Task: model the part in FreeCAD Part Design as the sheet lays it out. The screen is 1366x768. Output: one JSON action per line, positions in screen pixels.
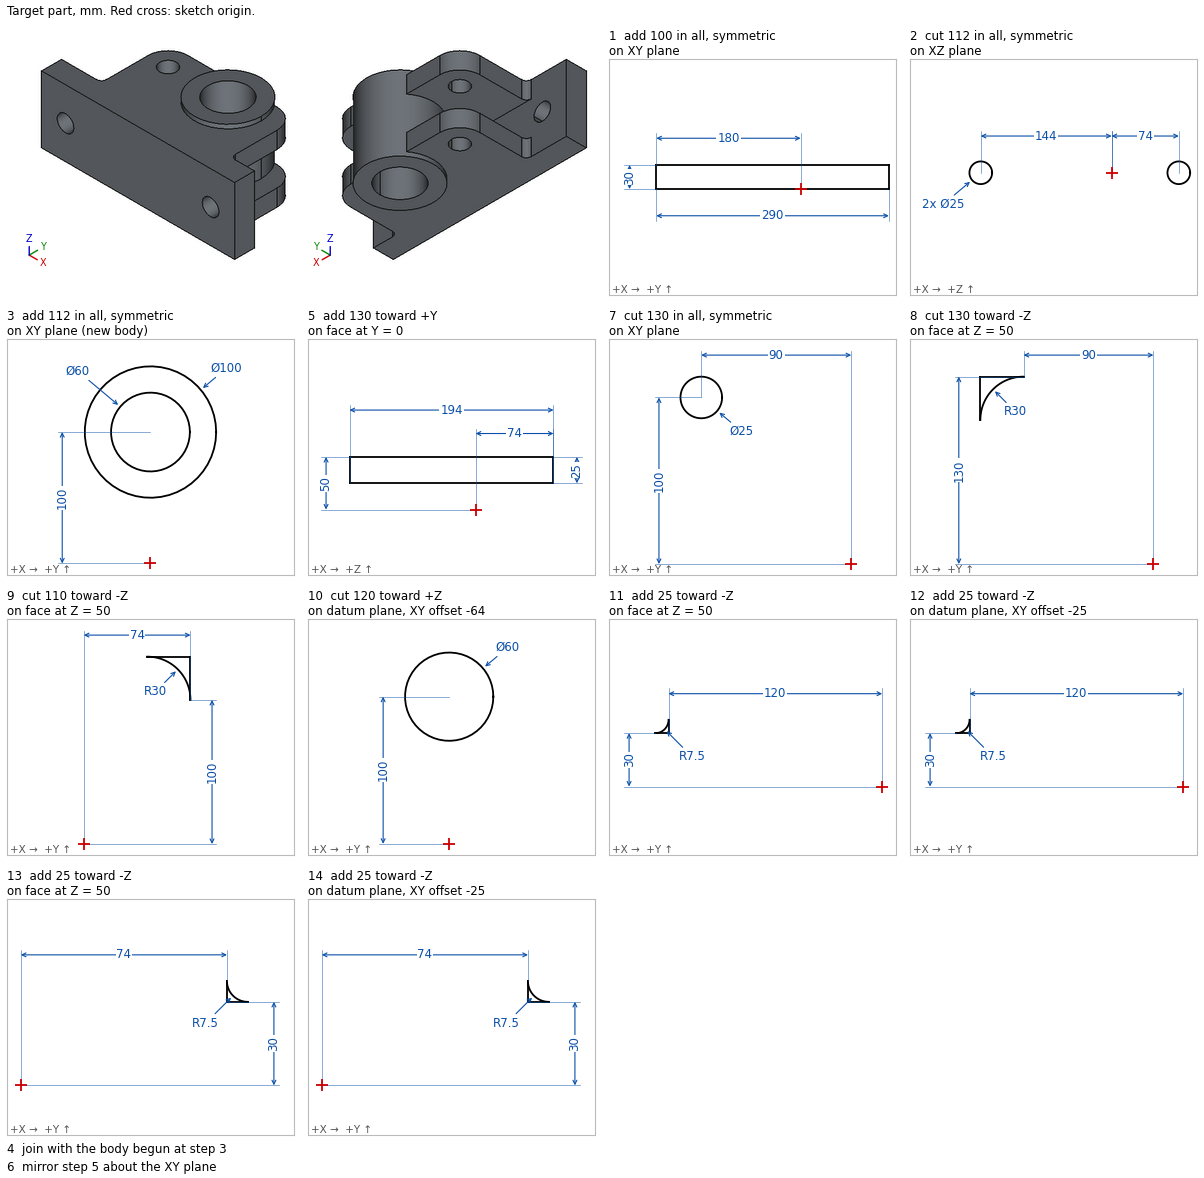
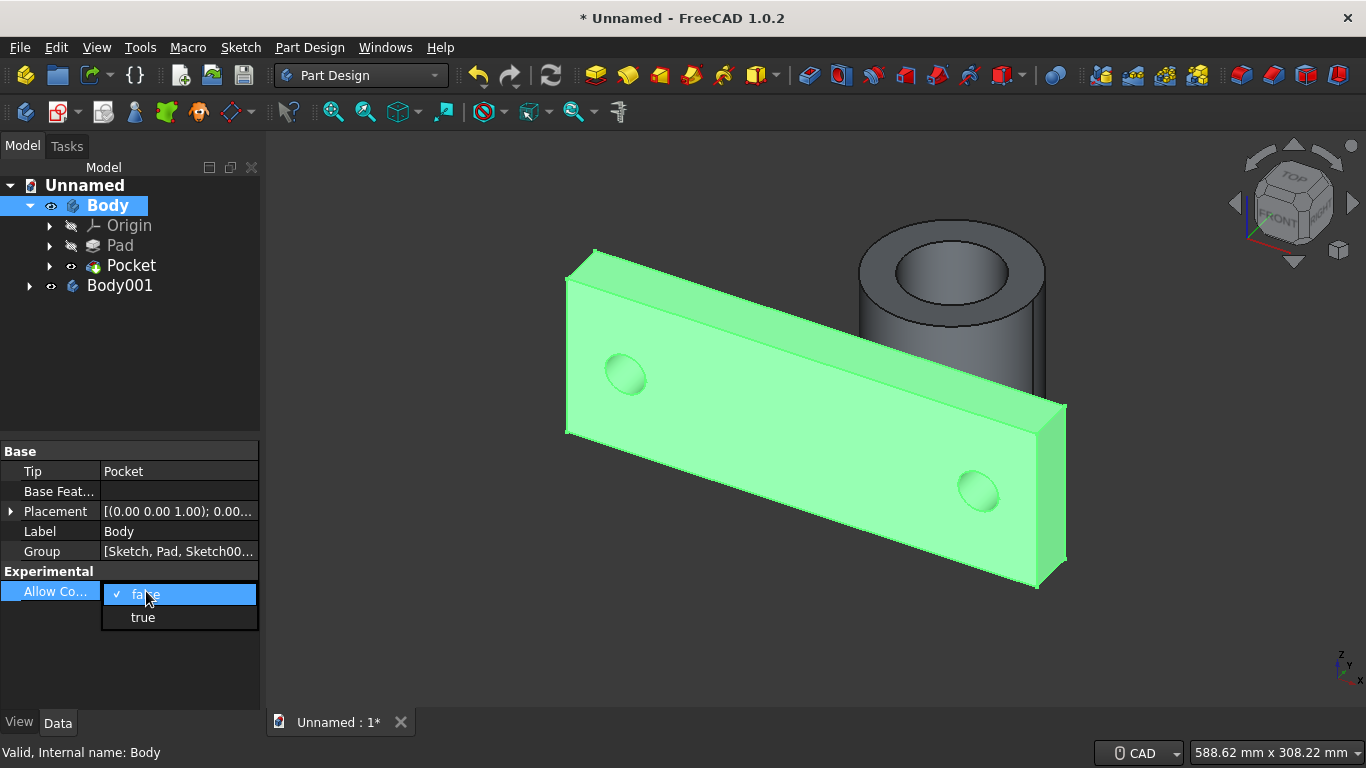
{"action": "left_click", "coordinate": [179, 618]}
{"action": "key", "text": "Return"}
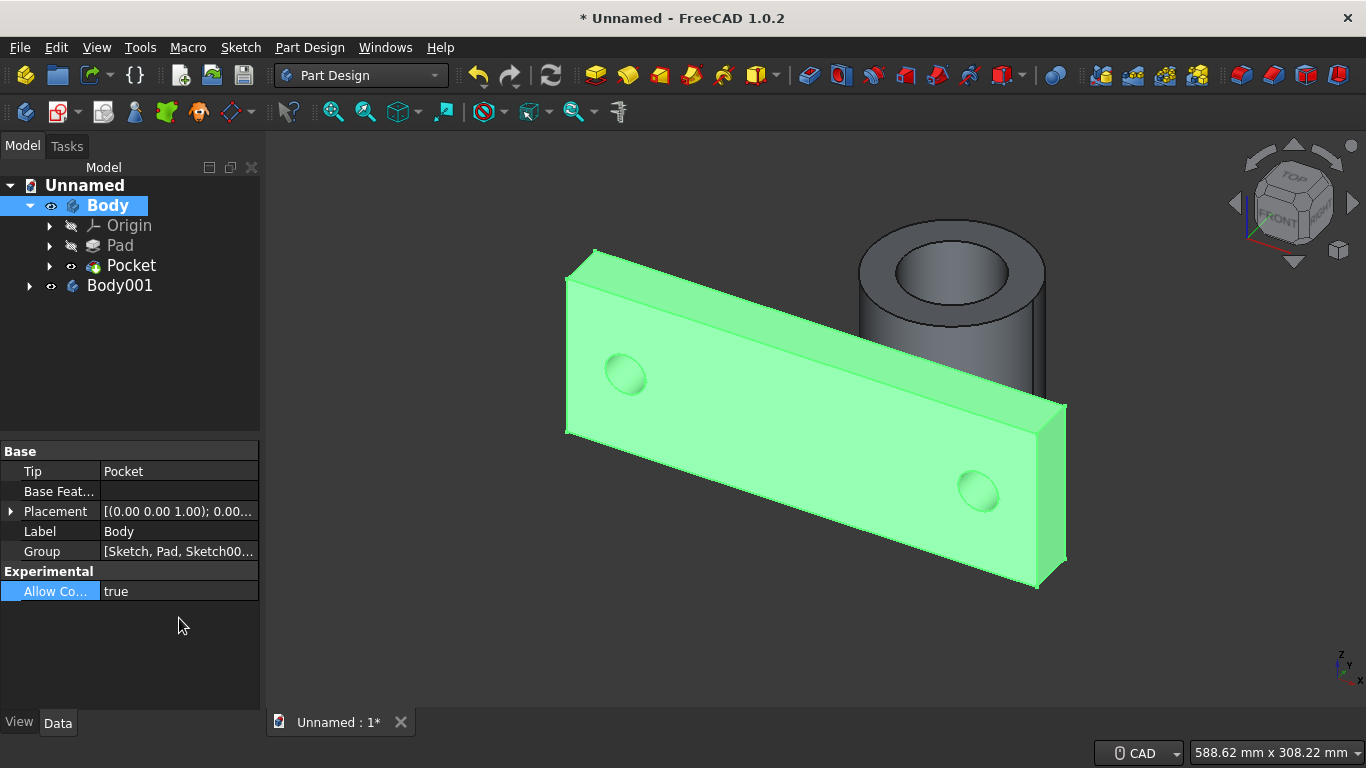
{"action": "left_click", "coordinate": [96, 286]}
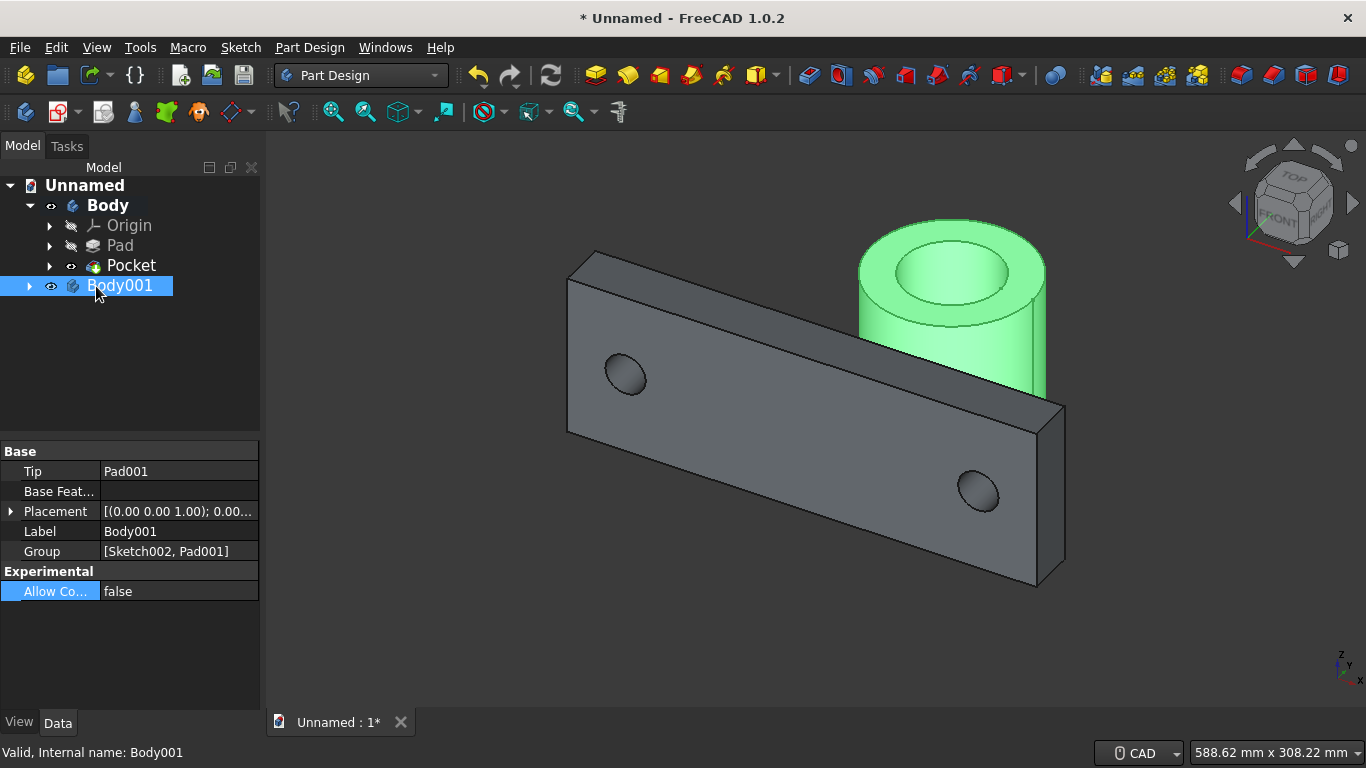
{"action": "left_click", "coordinate": [1056, 76]}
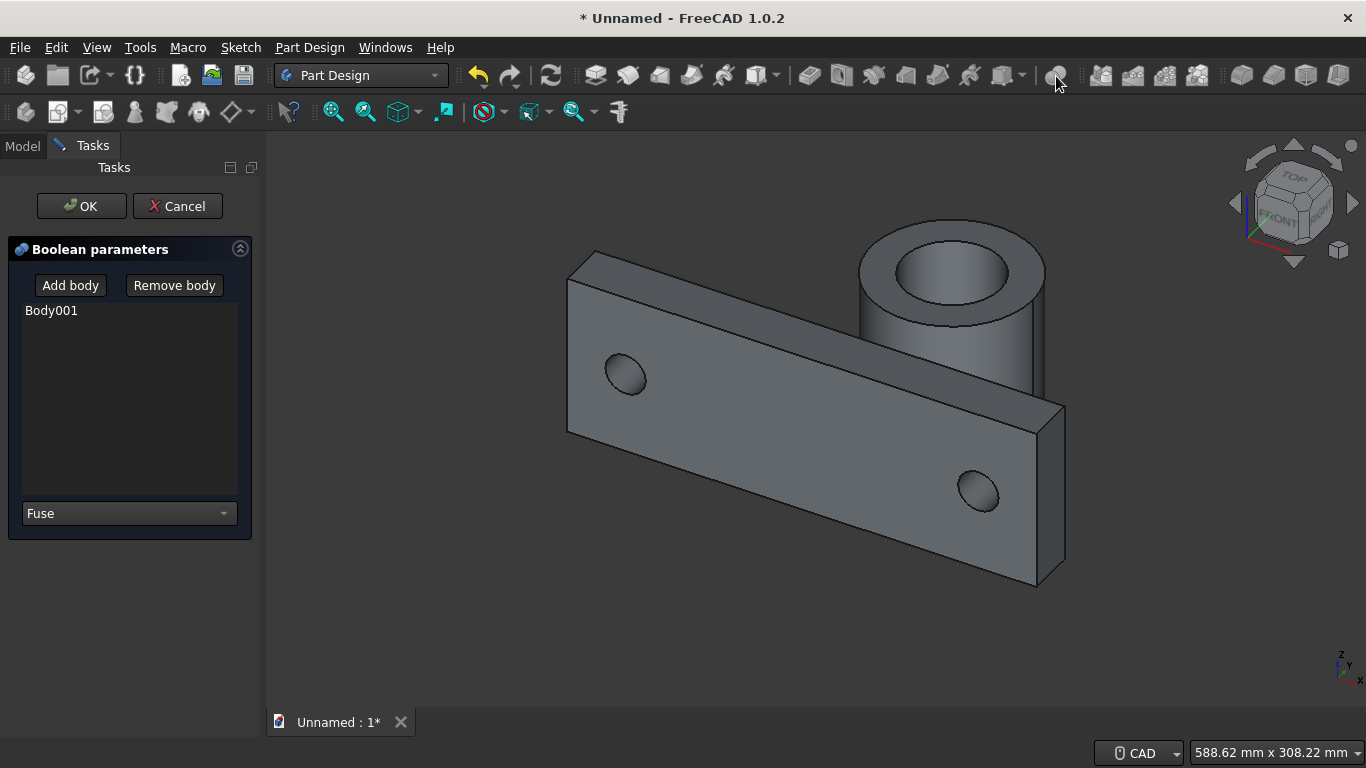
{"action": "left_click", "coordinate": [82, 206]}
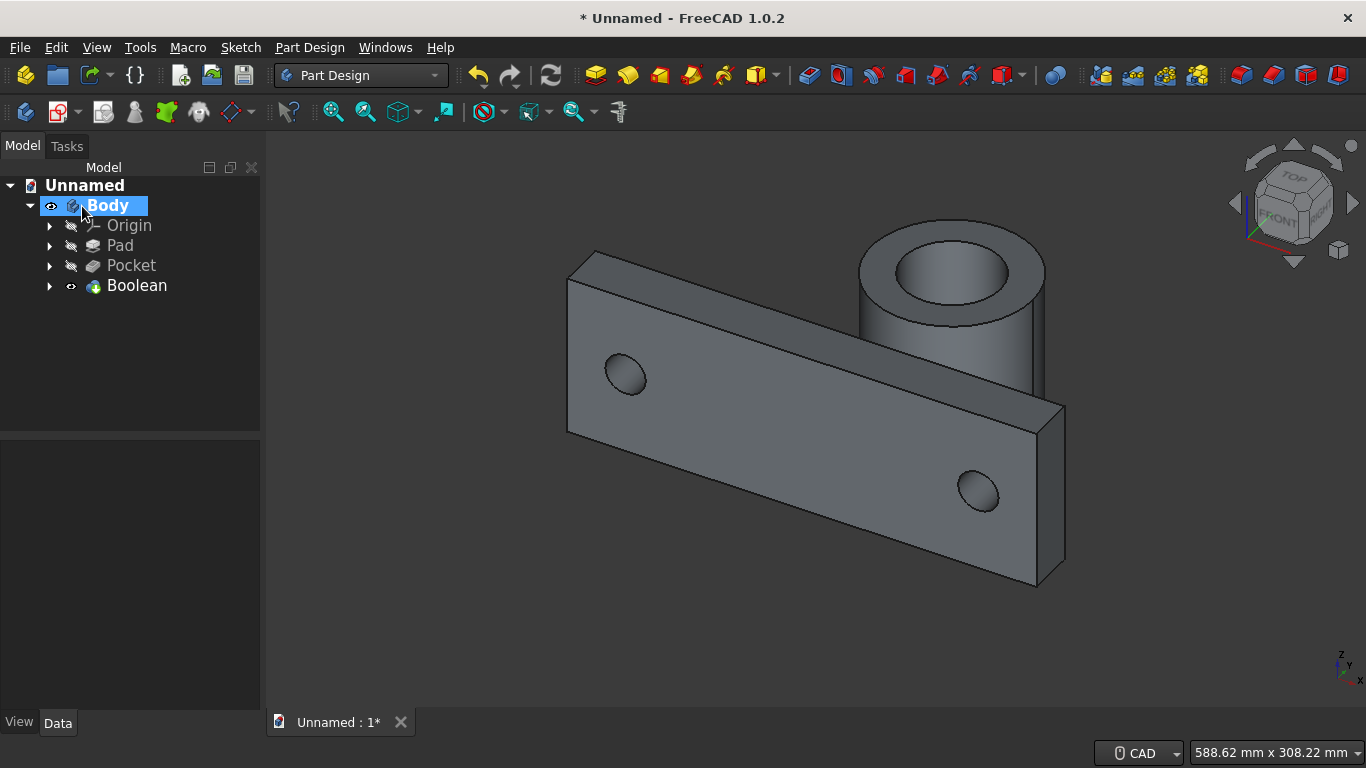
{"action": "left_click", "coordinate": [334, 112]}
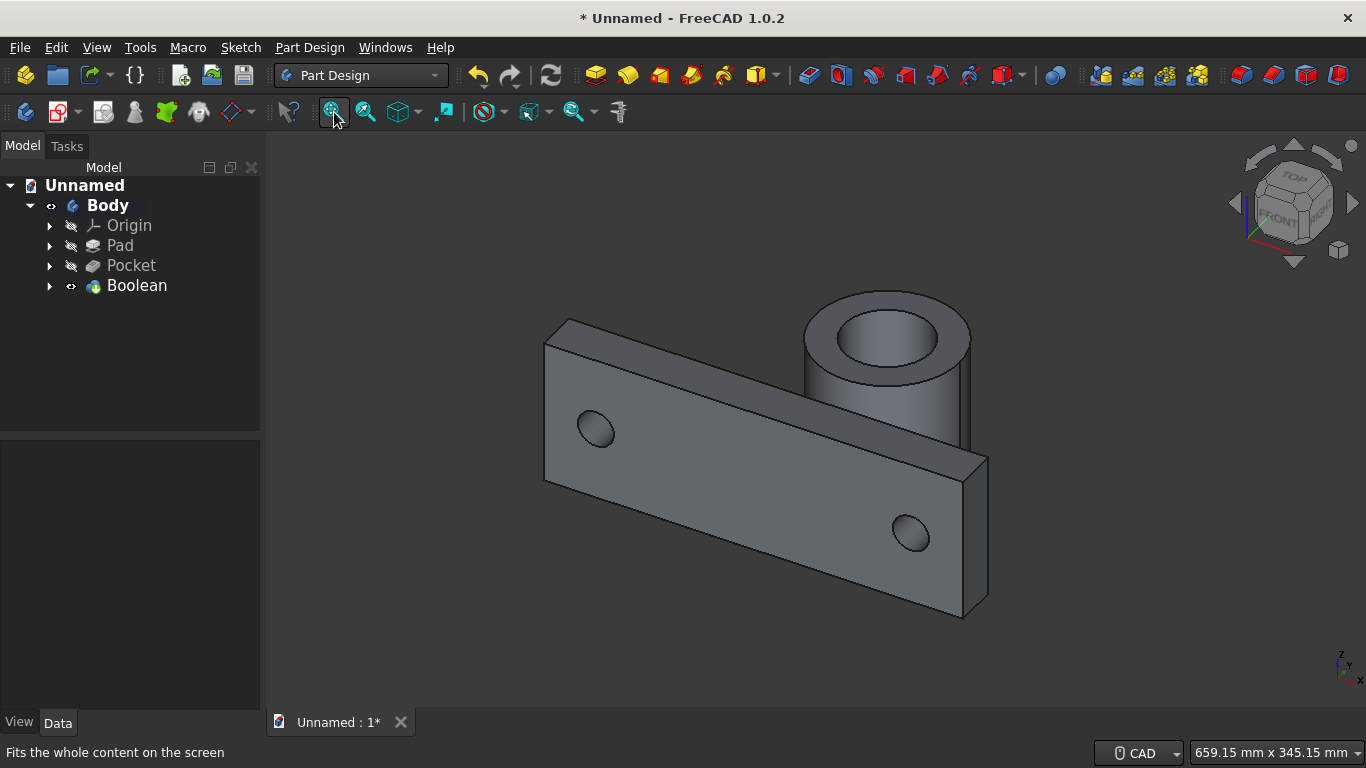
{"action": "left_click", "coordinate": [813, 500]}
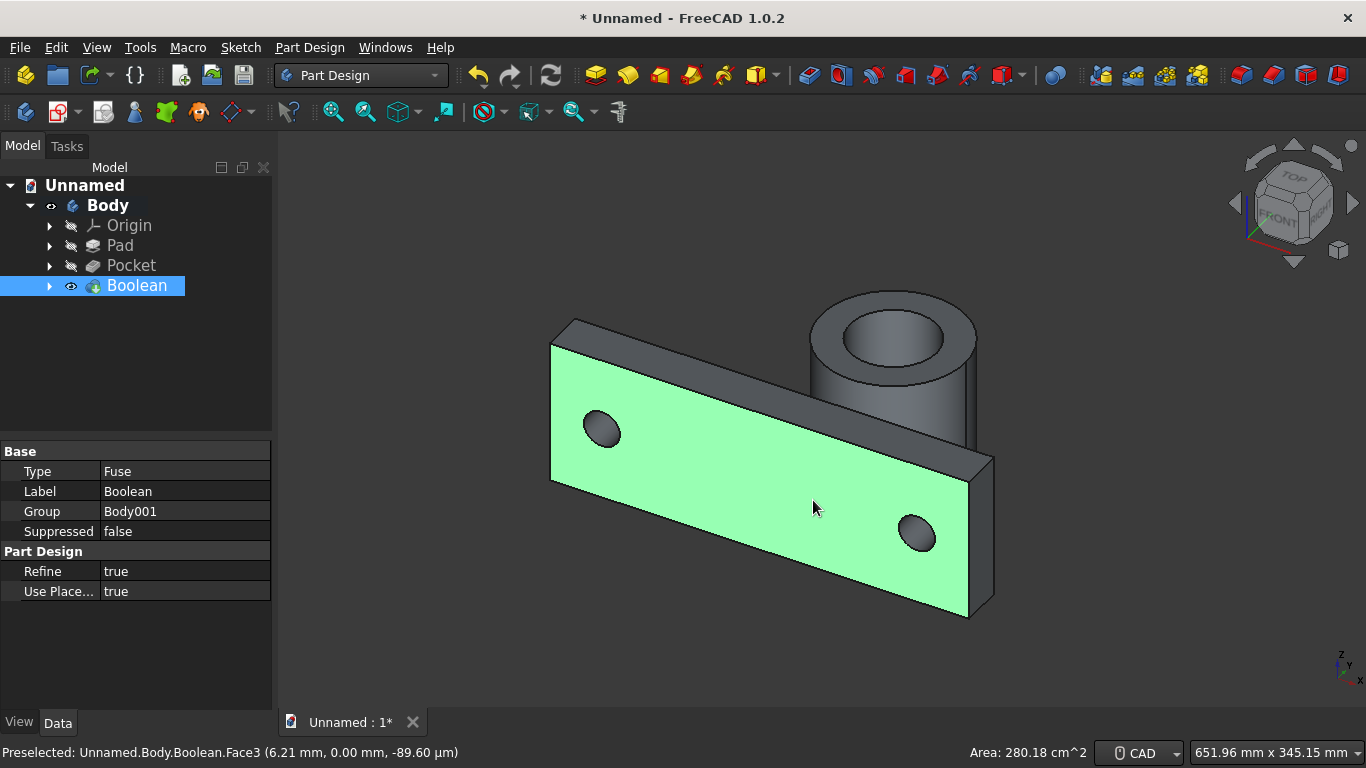
{"action": "left_click", "coordinate": [58, 112]}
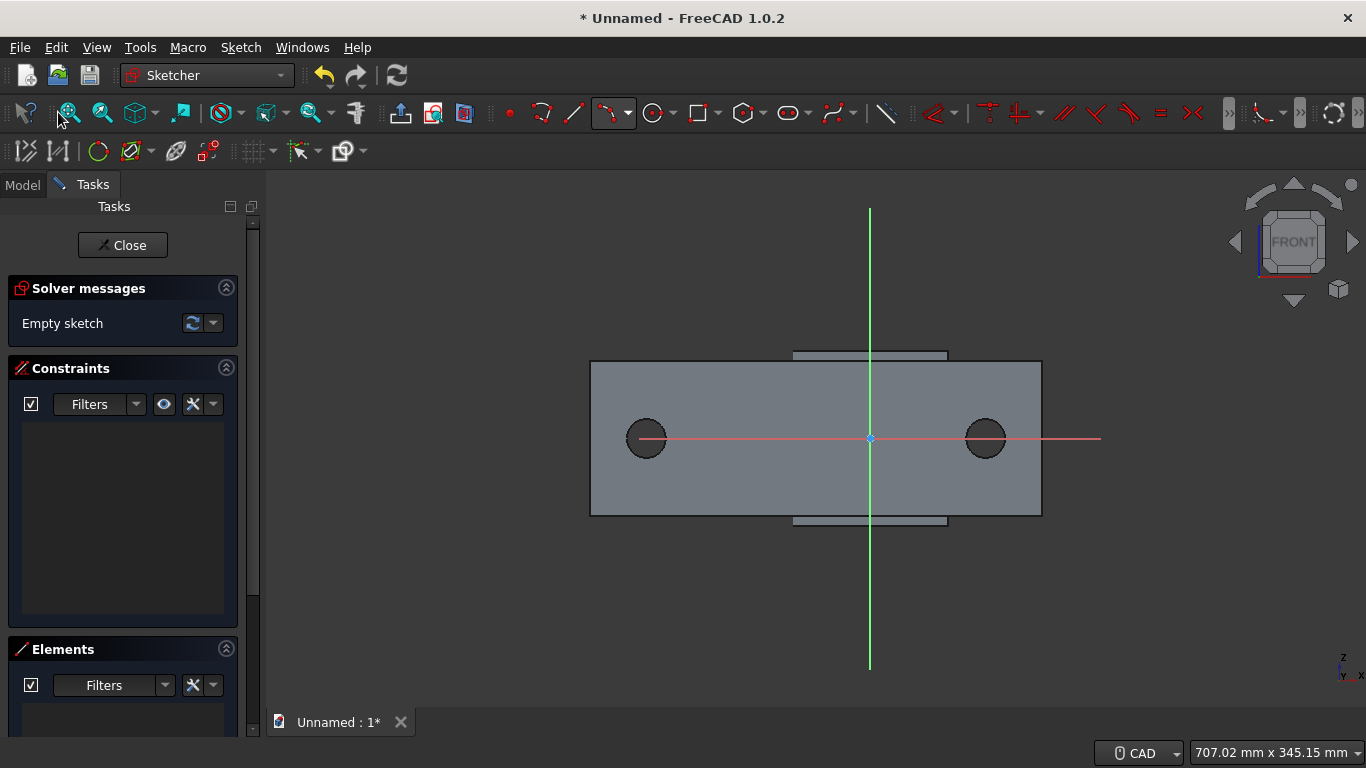
{"action": "scroll", "coordinate": [906, 368], "scroll_direction": "up", "scroll_amount": 4}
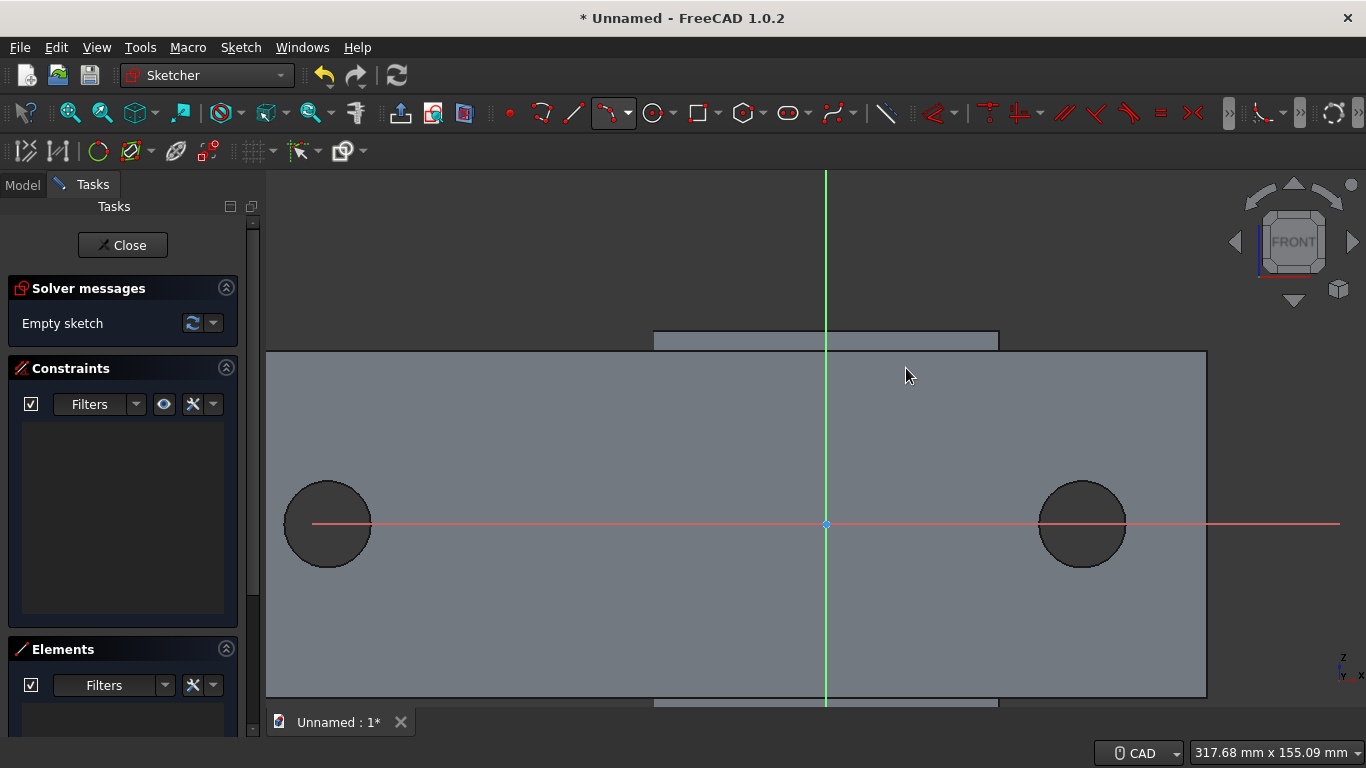
{"action": "left_click", "coordinate": [698, 114]}